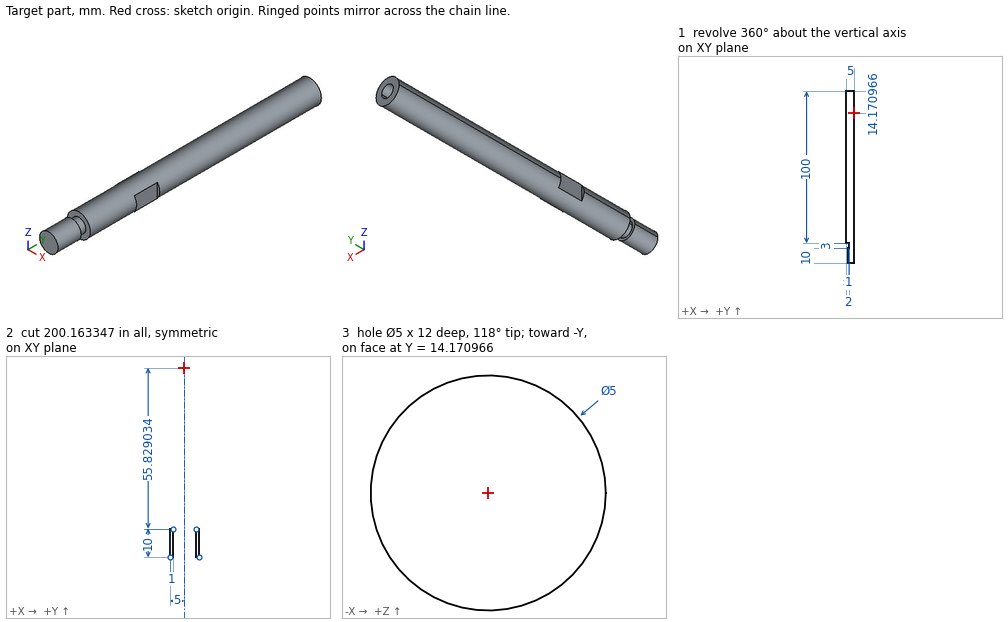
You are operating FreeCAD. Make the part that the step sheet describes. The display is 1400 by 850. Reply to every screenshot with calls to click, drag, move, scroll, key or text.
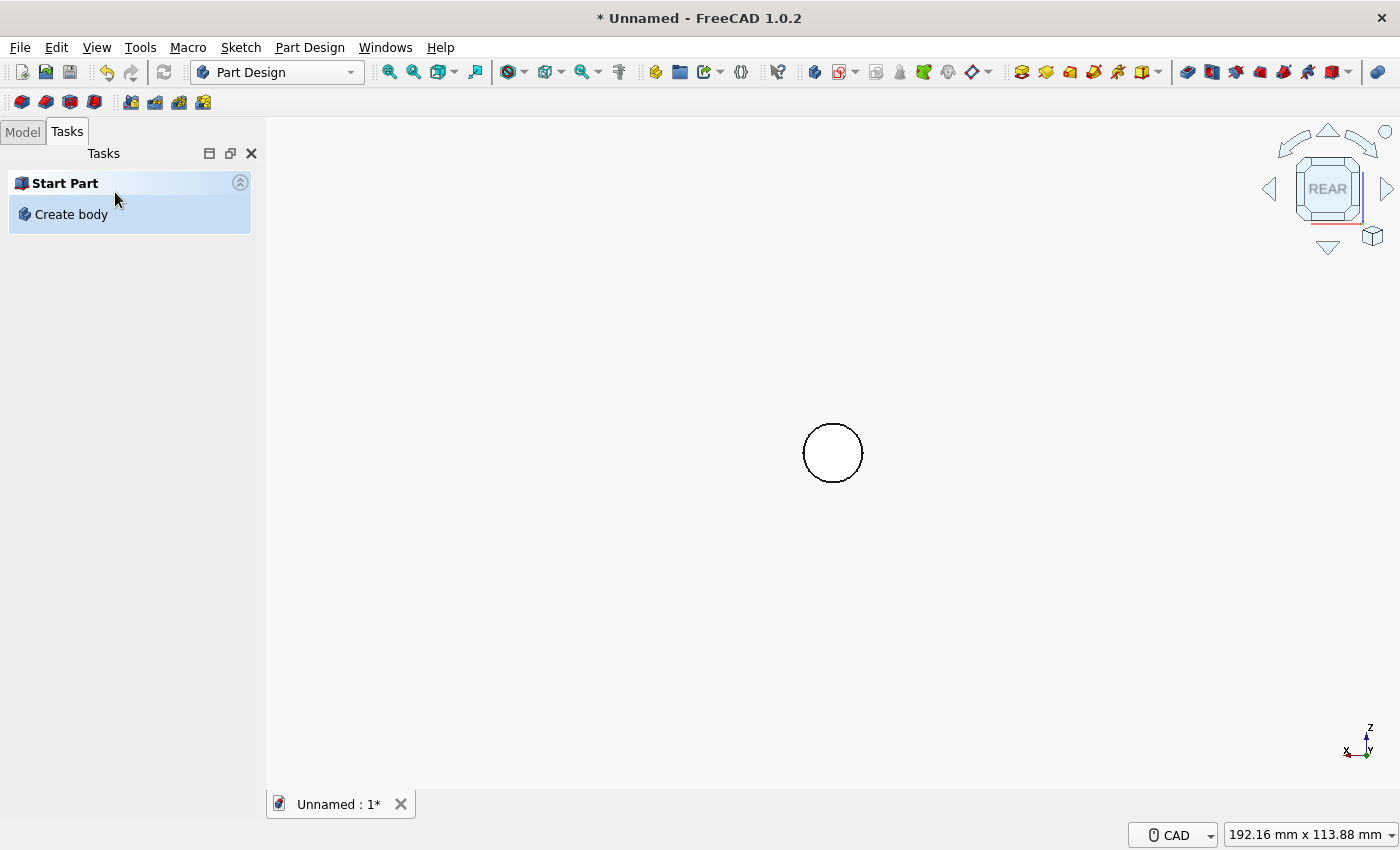
click(390, 72)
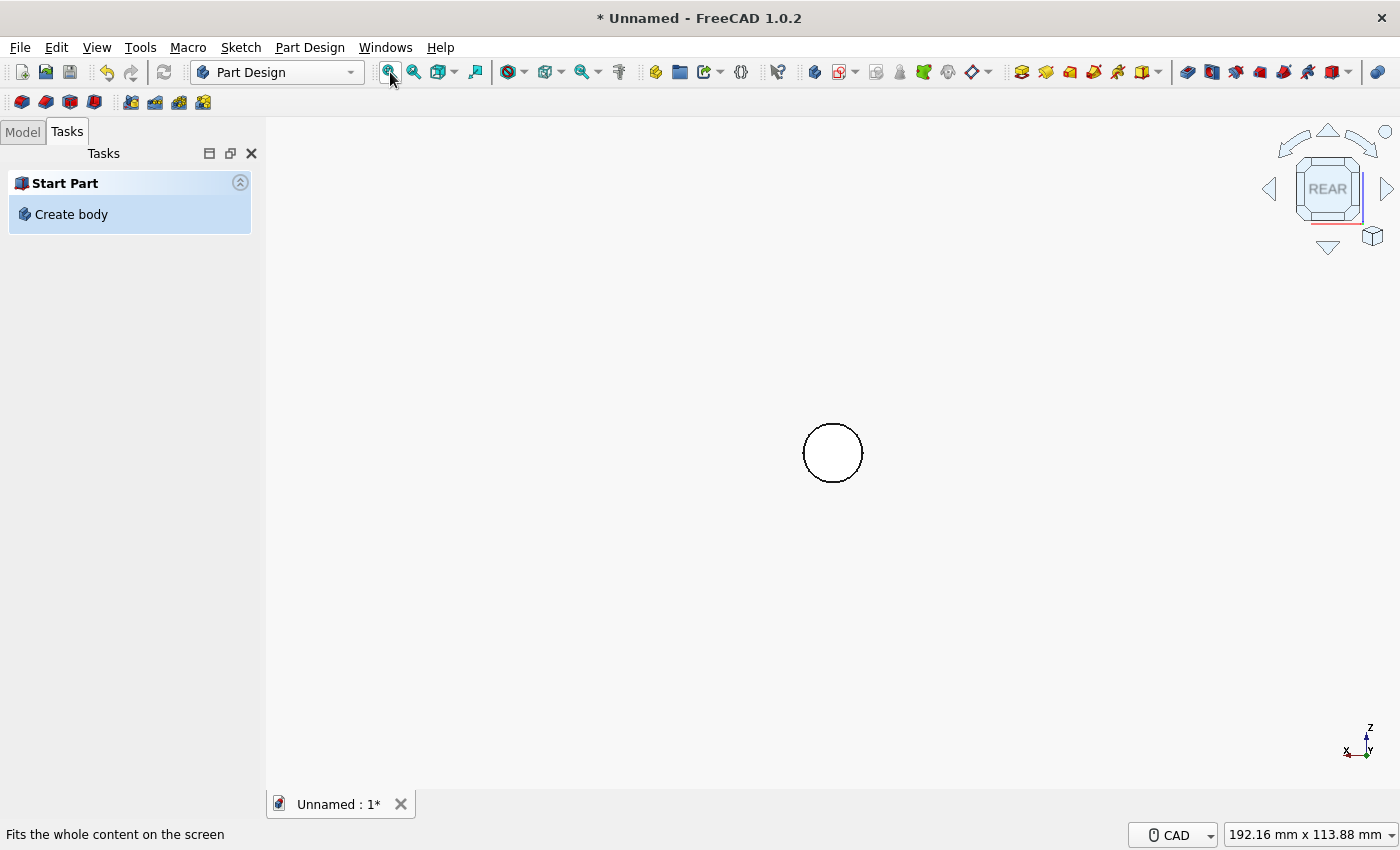
click(833, 452)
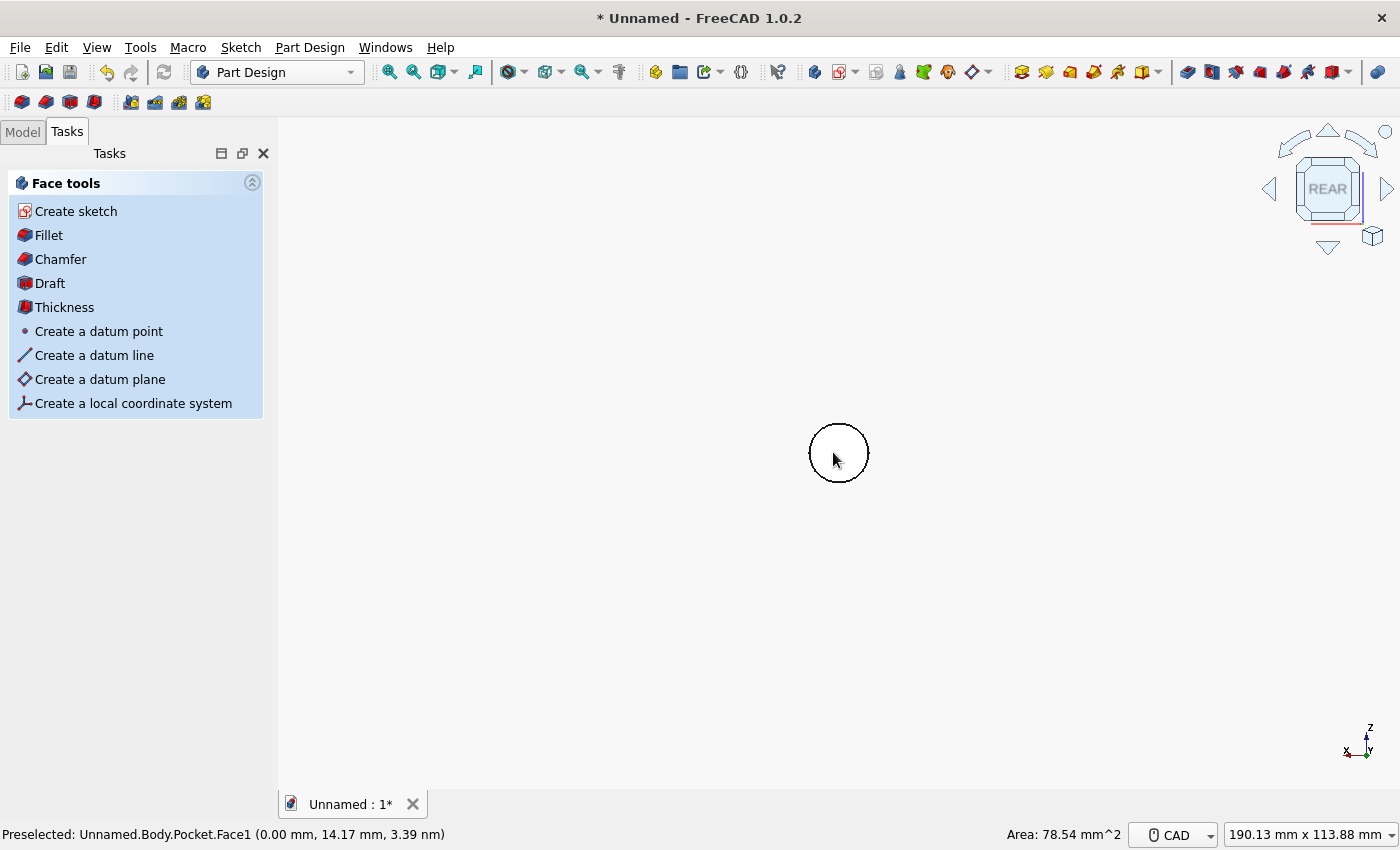
click(840, 72)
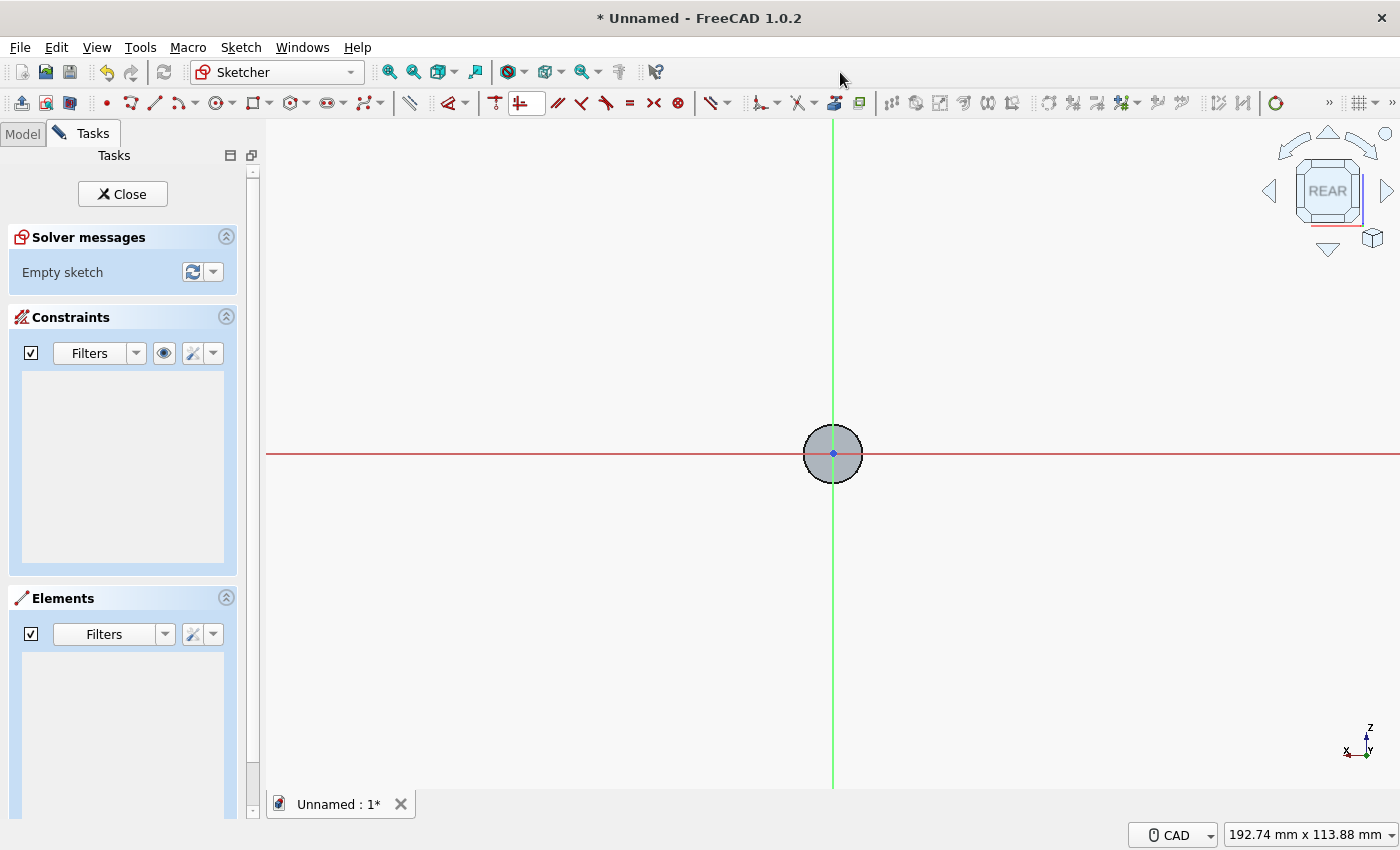
scroll(838, 454, up, 13)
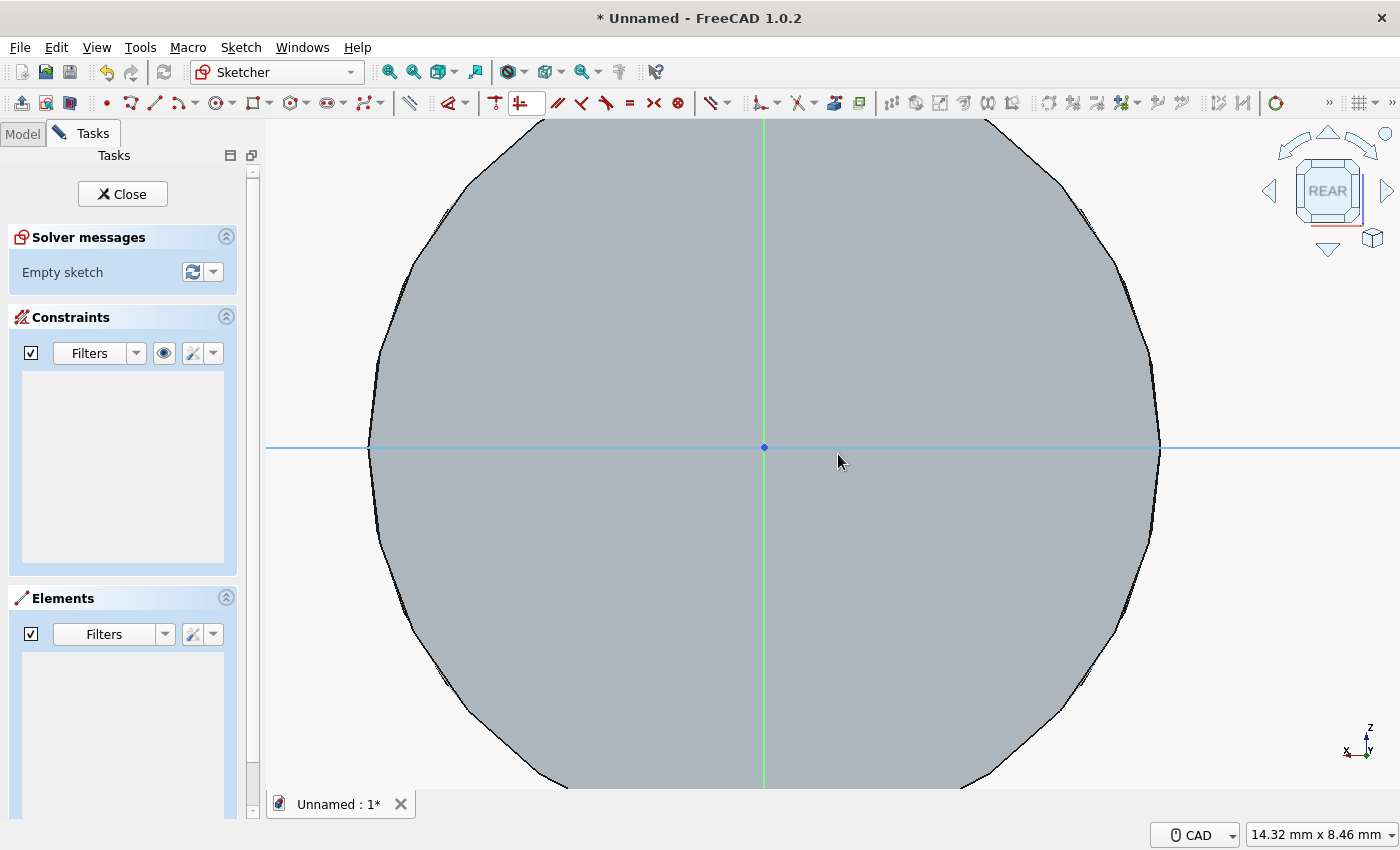
click(216, 104)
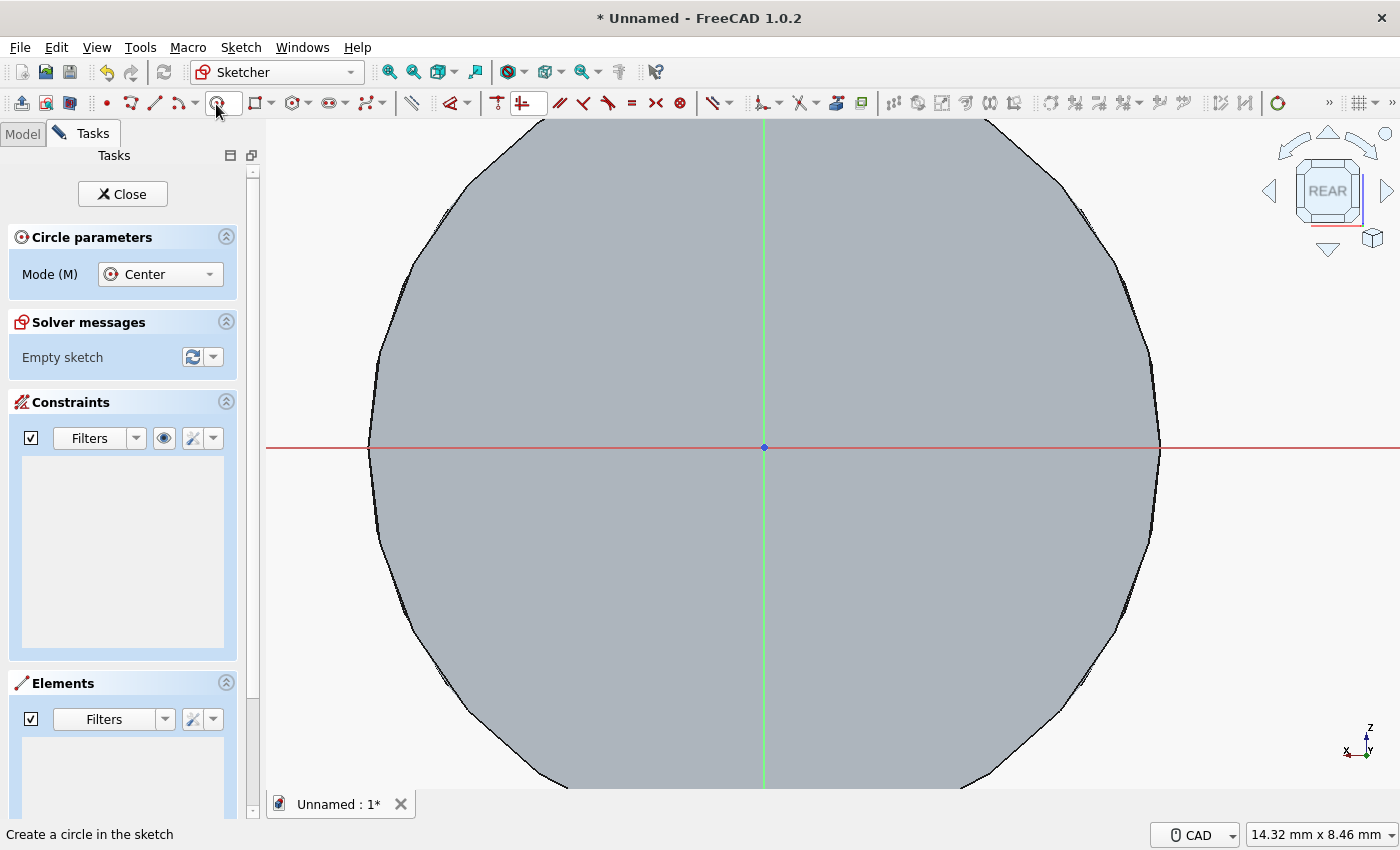
click(764, 448)
click(904, 308)
key(Escape)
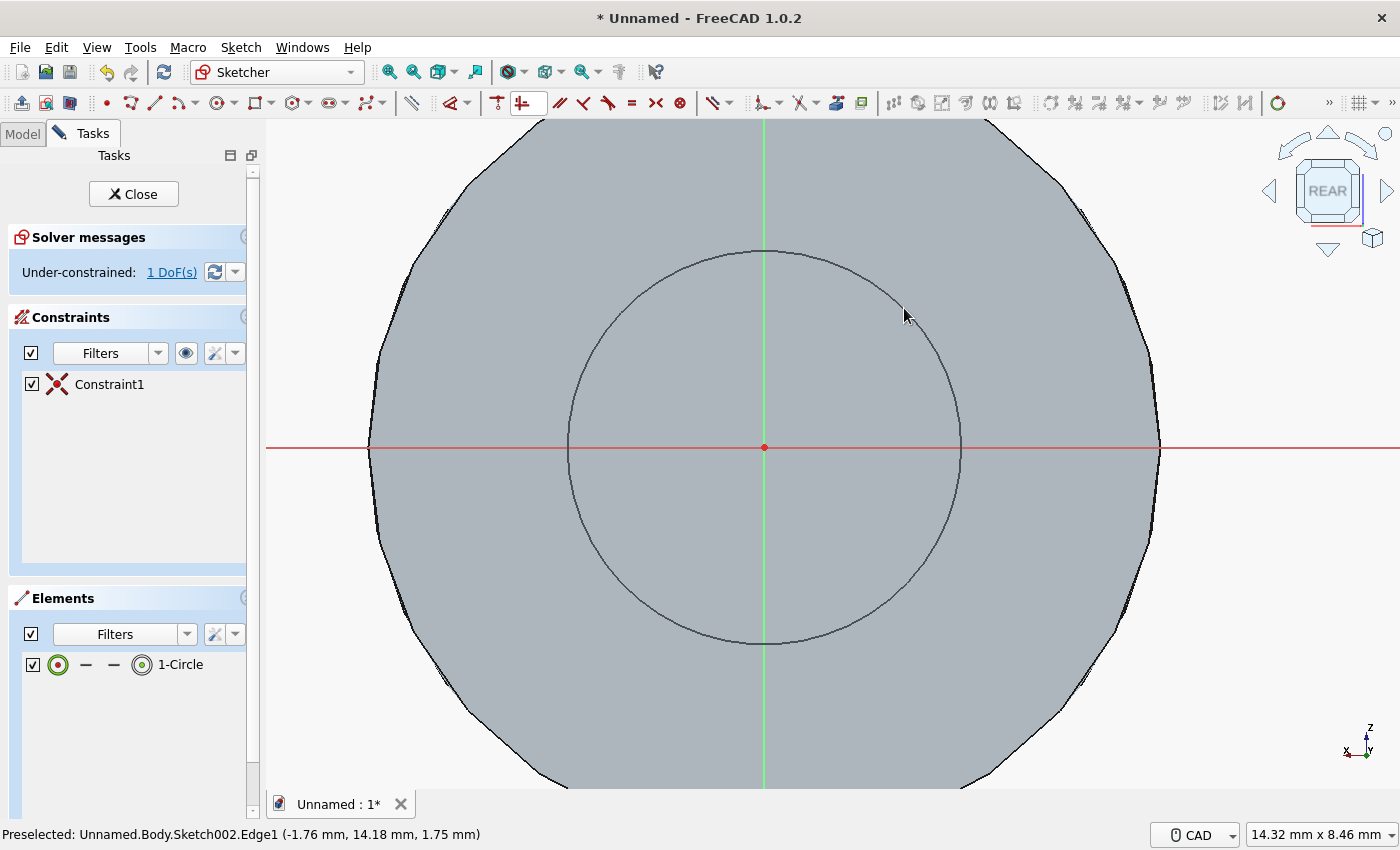
click(450, 104)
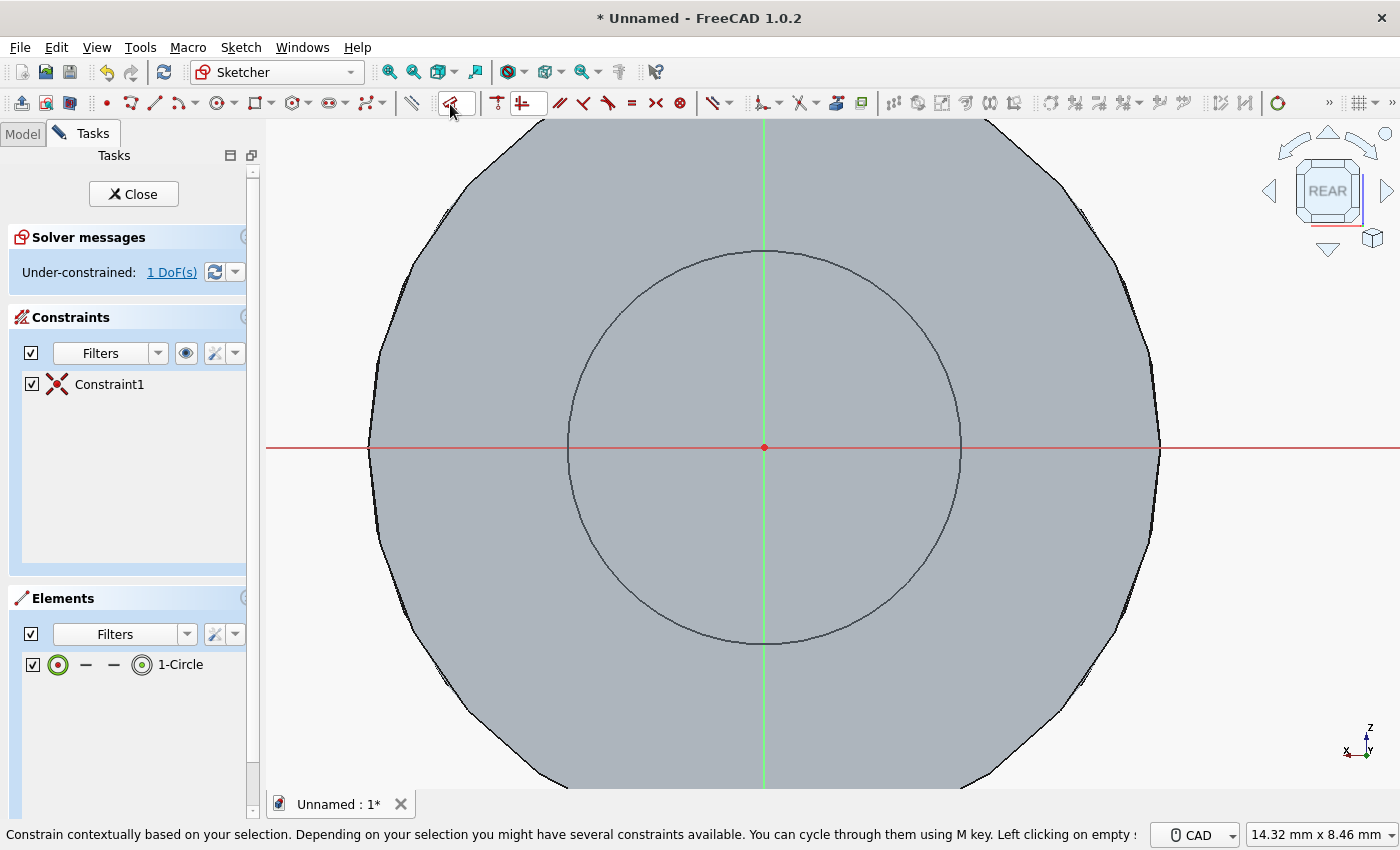
click(903, 308)
click(926, 285)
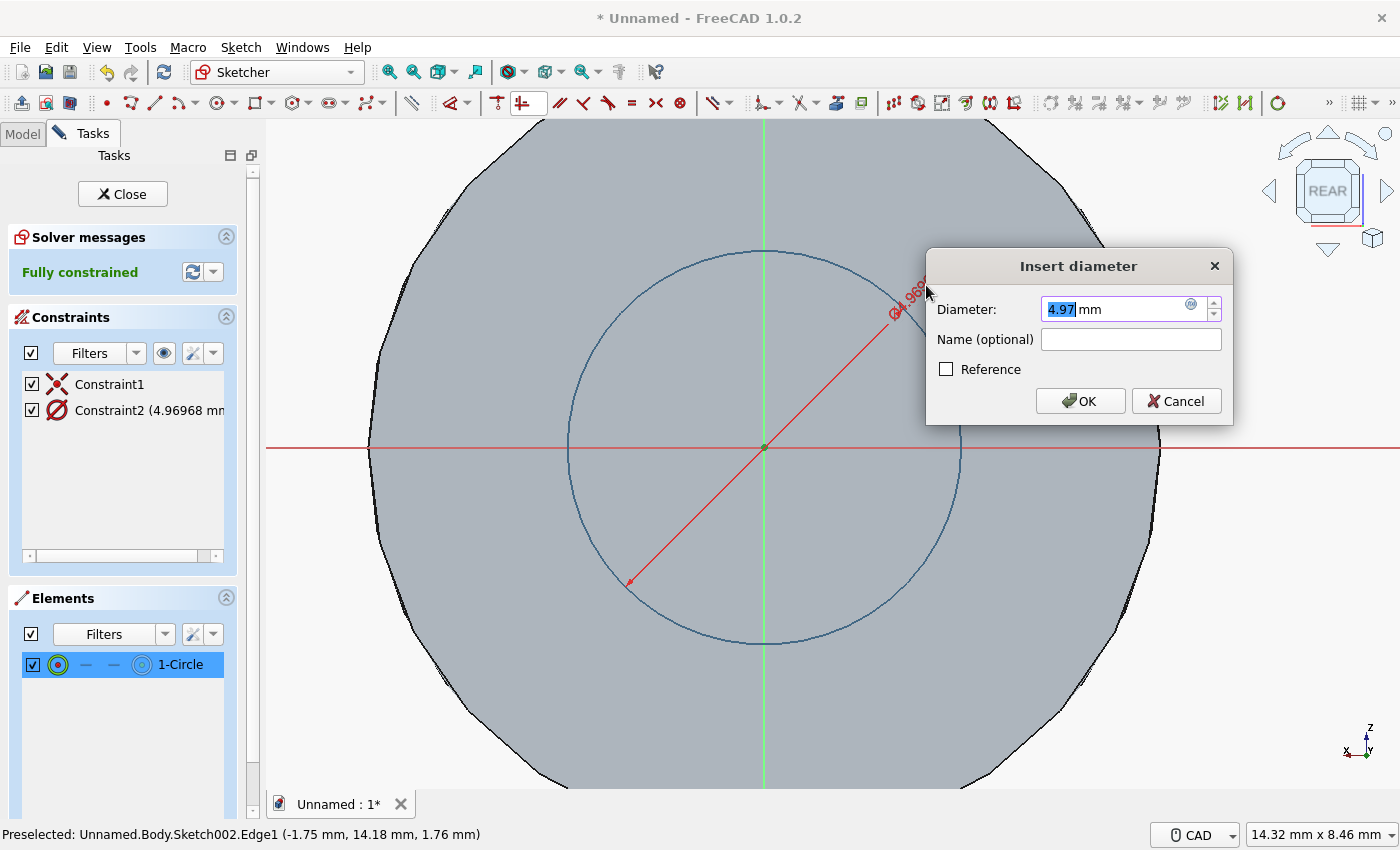
text(5)
key(Return)
key(Escape)